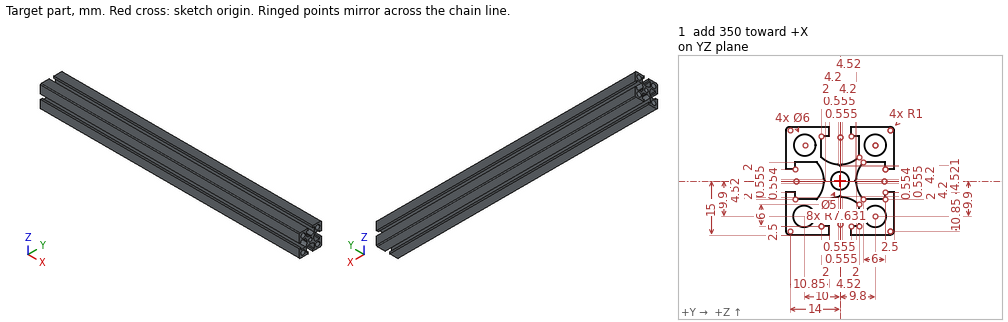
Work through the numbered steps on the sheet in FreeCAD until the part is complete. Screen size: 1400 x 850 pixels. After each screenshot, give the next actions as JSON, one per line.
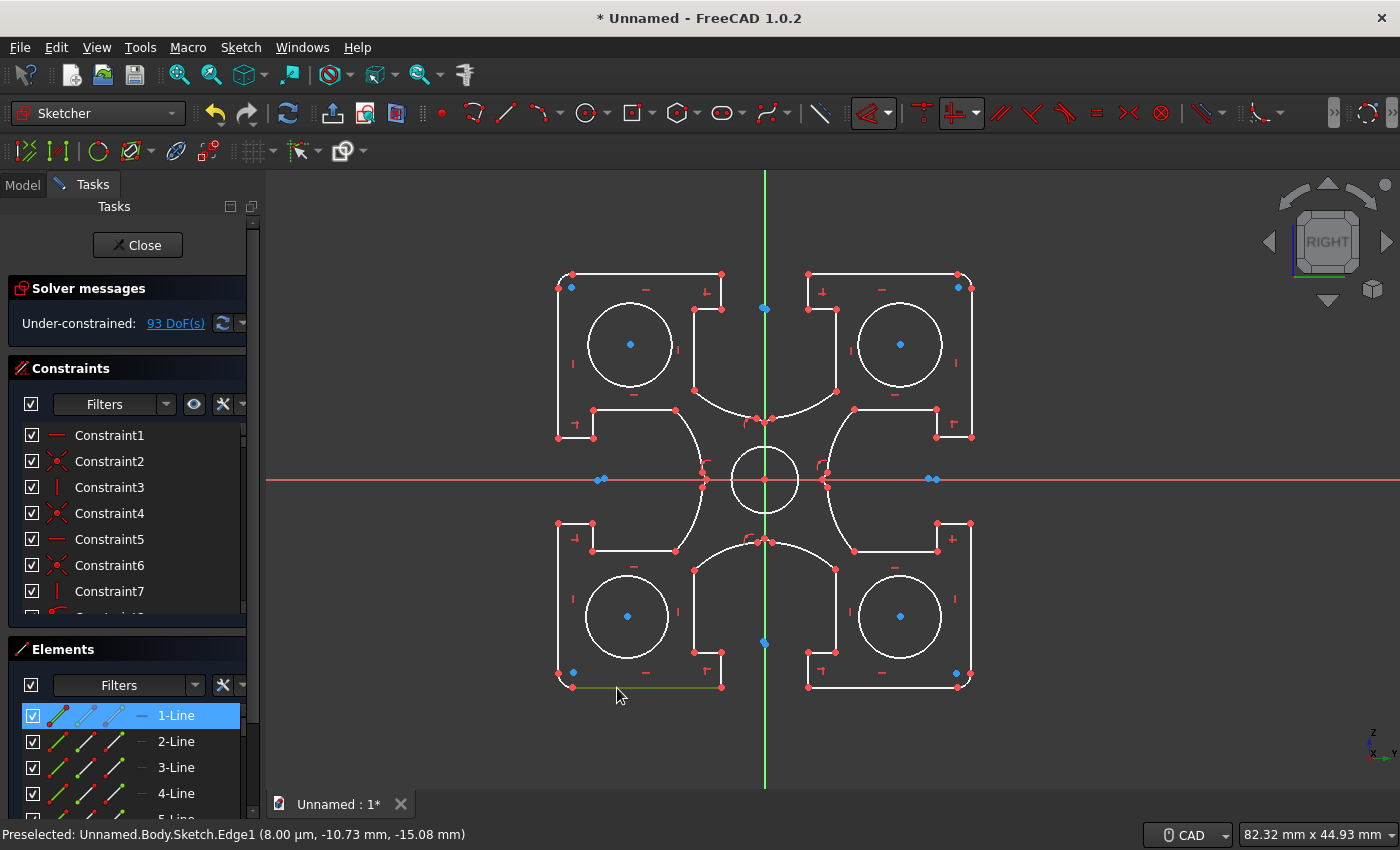
{"action": "scroll", "coordinate": [563, 683], "scroll_direction": "up", "scroll_amount": 2}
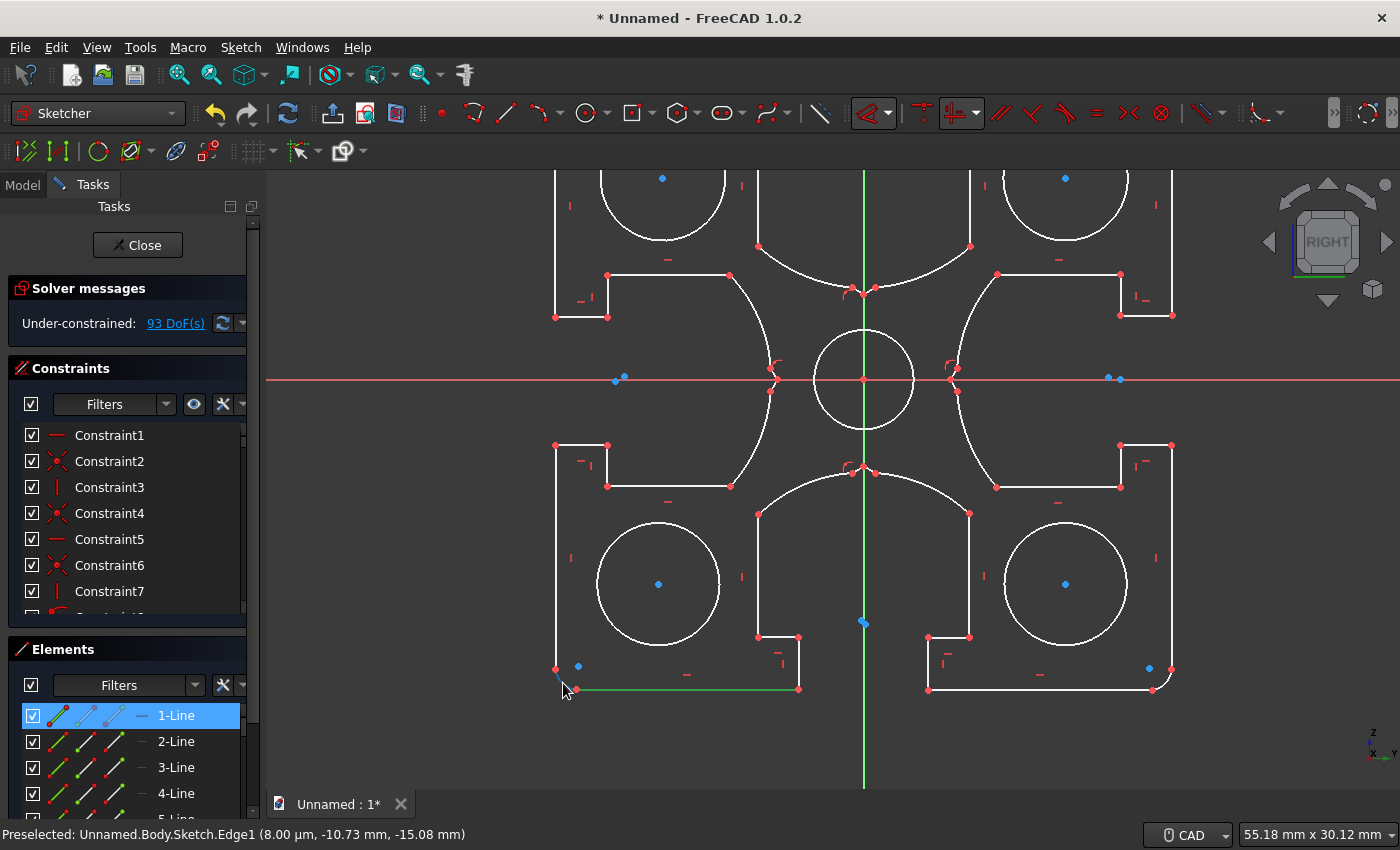
{"action": "left_click", "coordinate": [562, 683]}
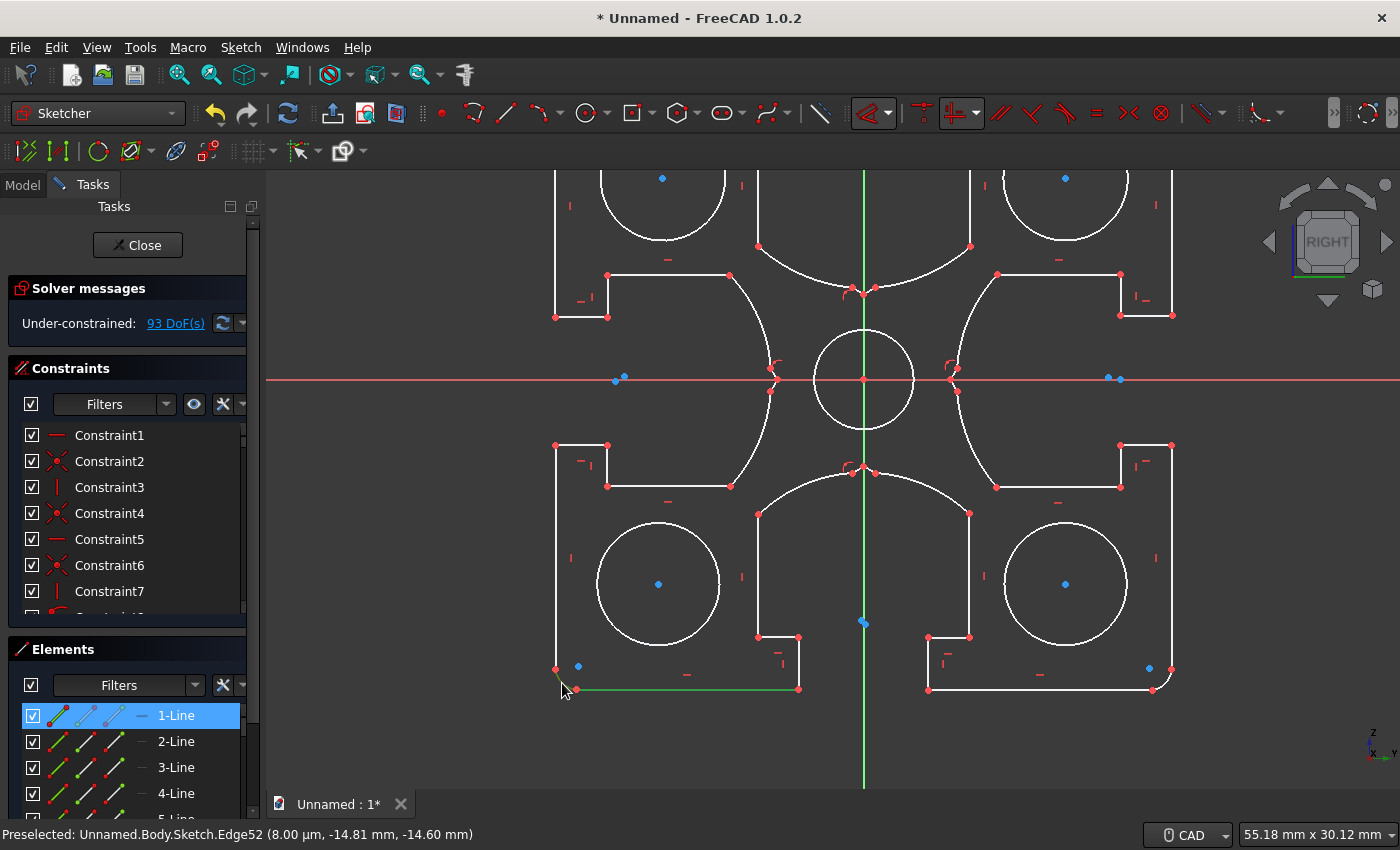
{"action": "left_click", "coordinate": [1066, 114]}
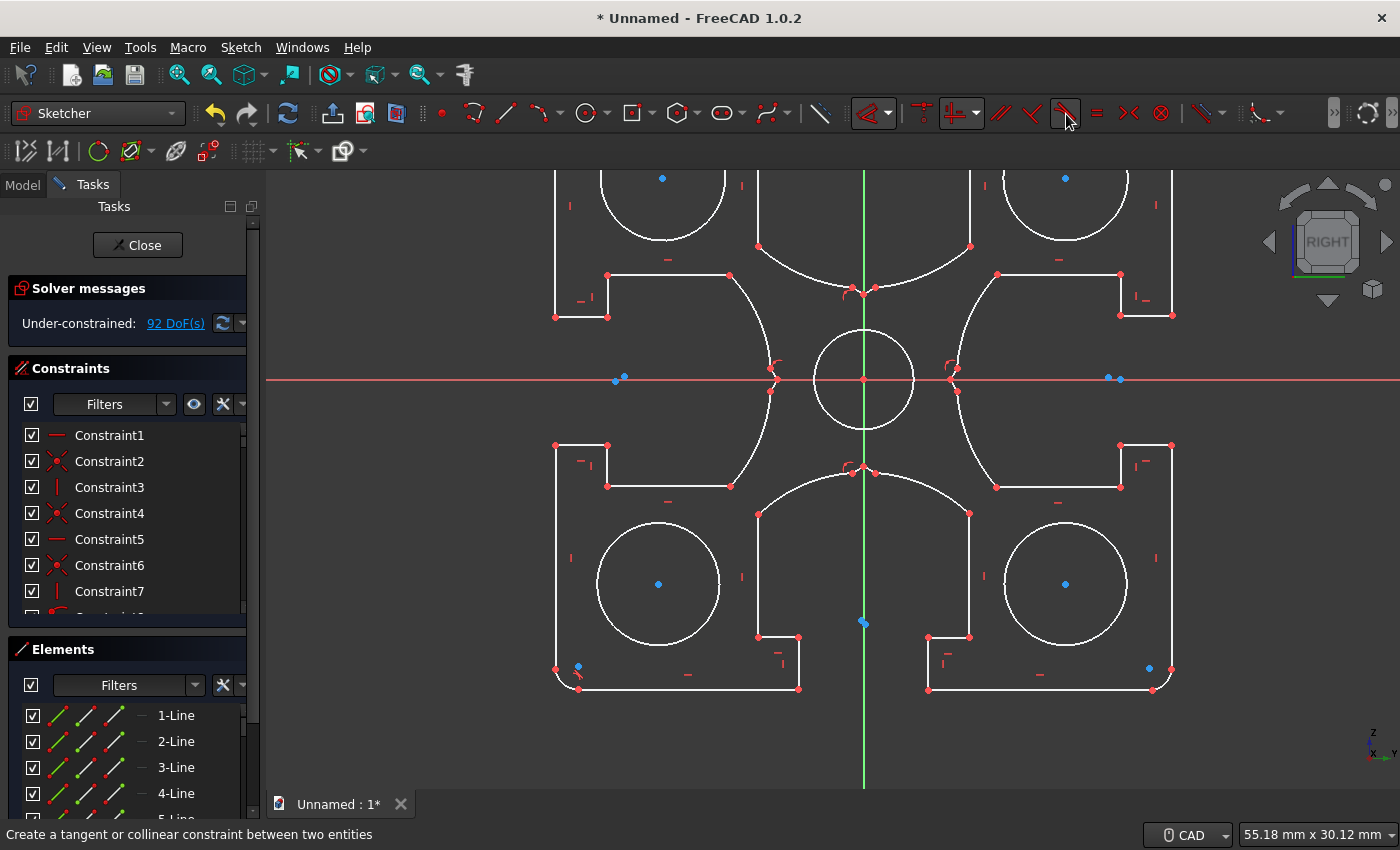
{"action": "left_click", "coordinate": [996, 690]}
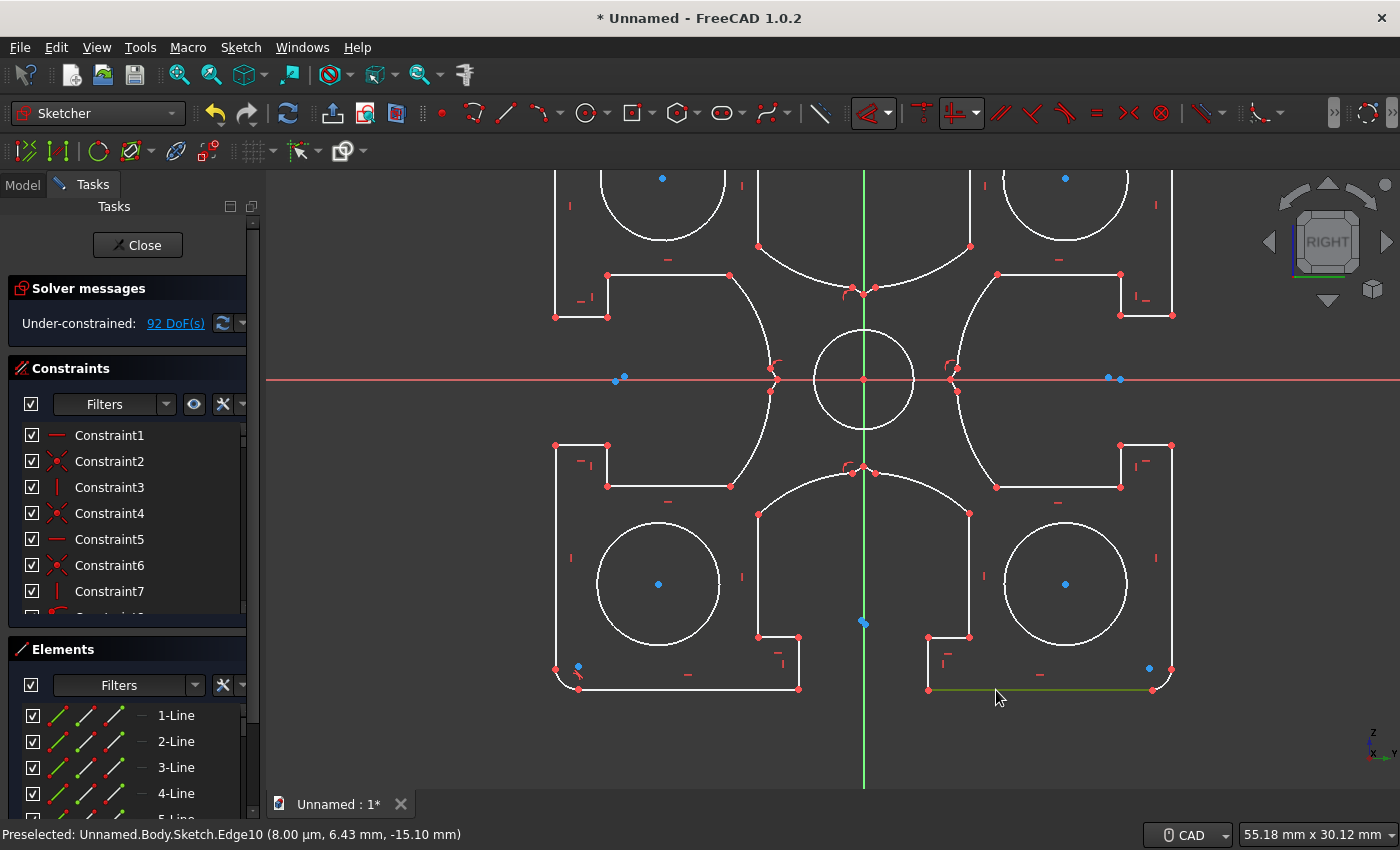
{"action": "scroll", "coordinate": [1161, 687], "scroll_direction": "up", "scroll_amount": 3}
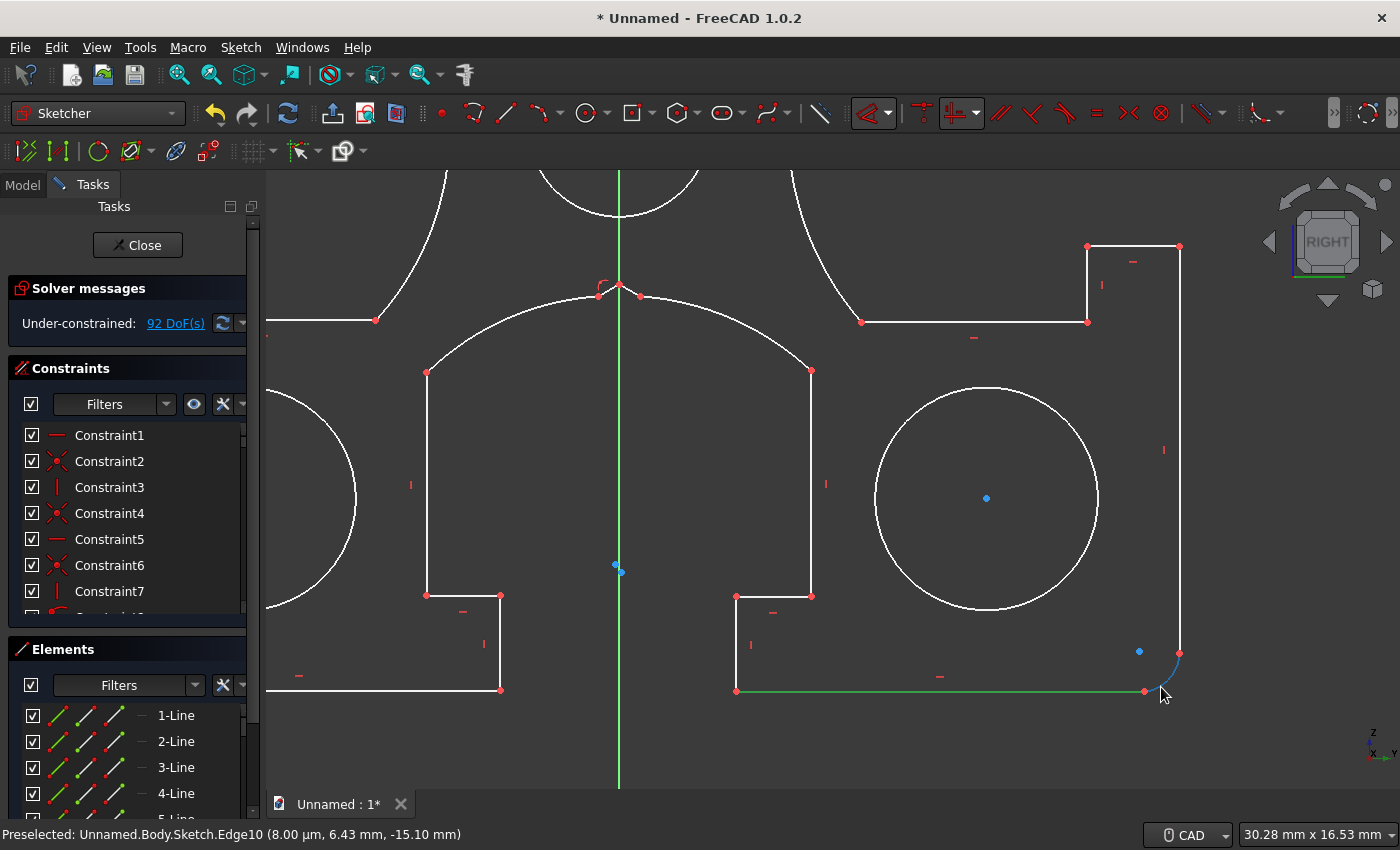
{"action": "left_click", "coordinate": [1160, 686]}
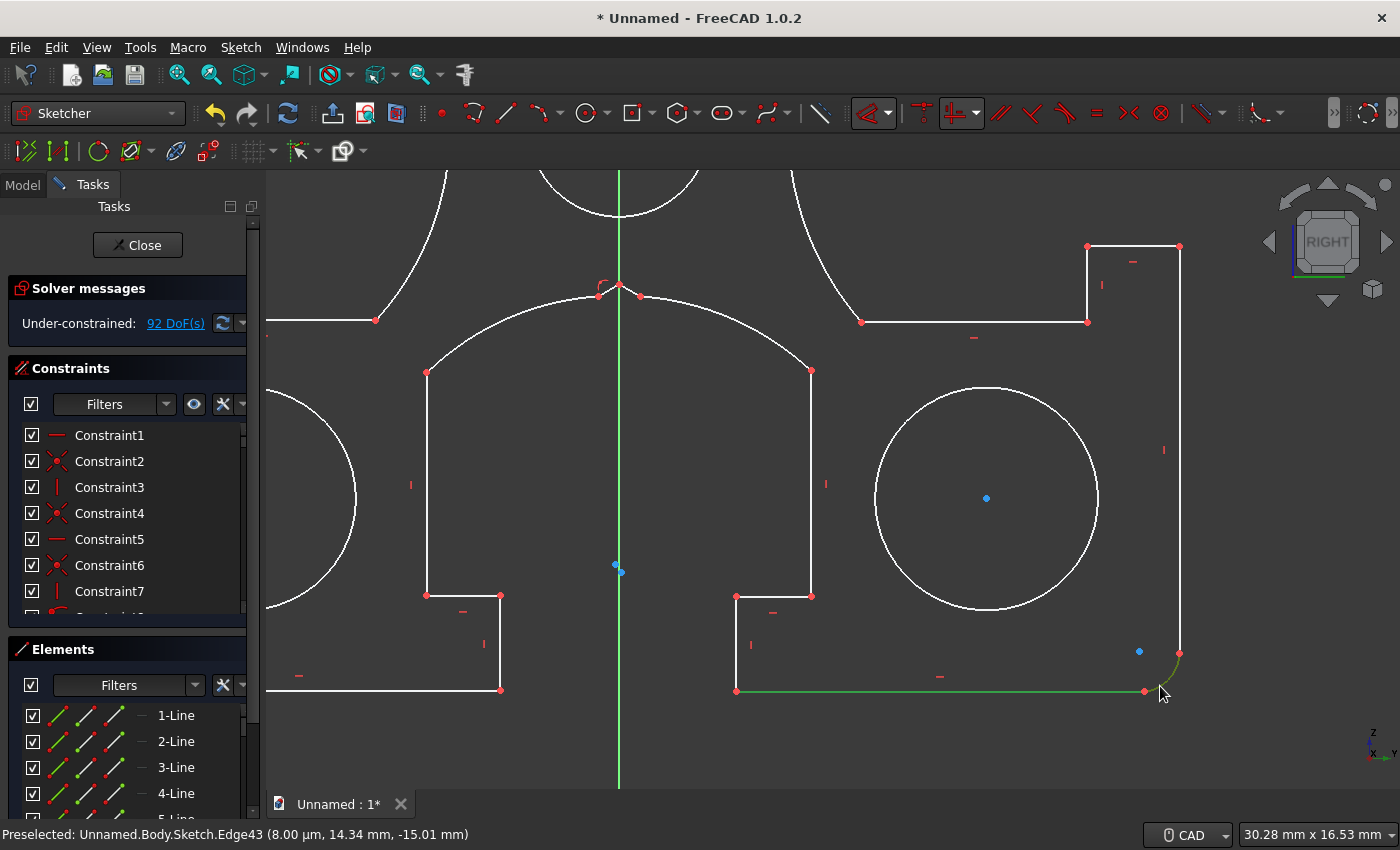
{"action": "left_click", "coordinate": [1066, 114]}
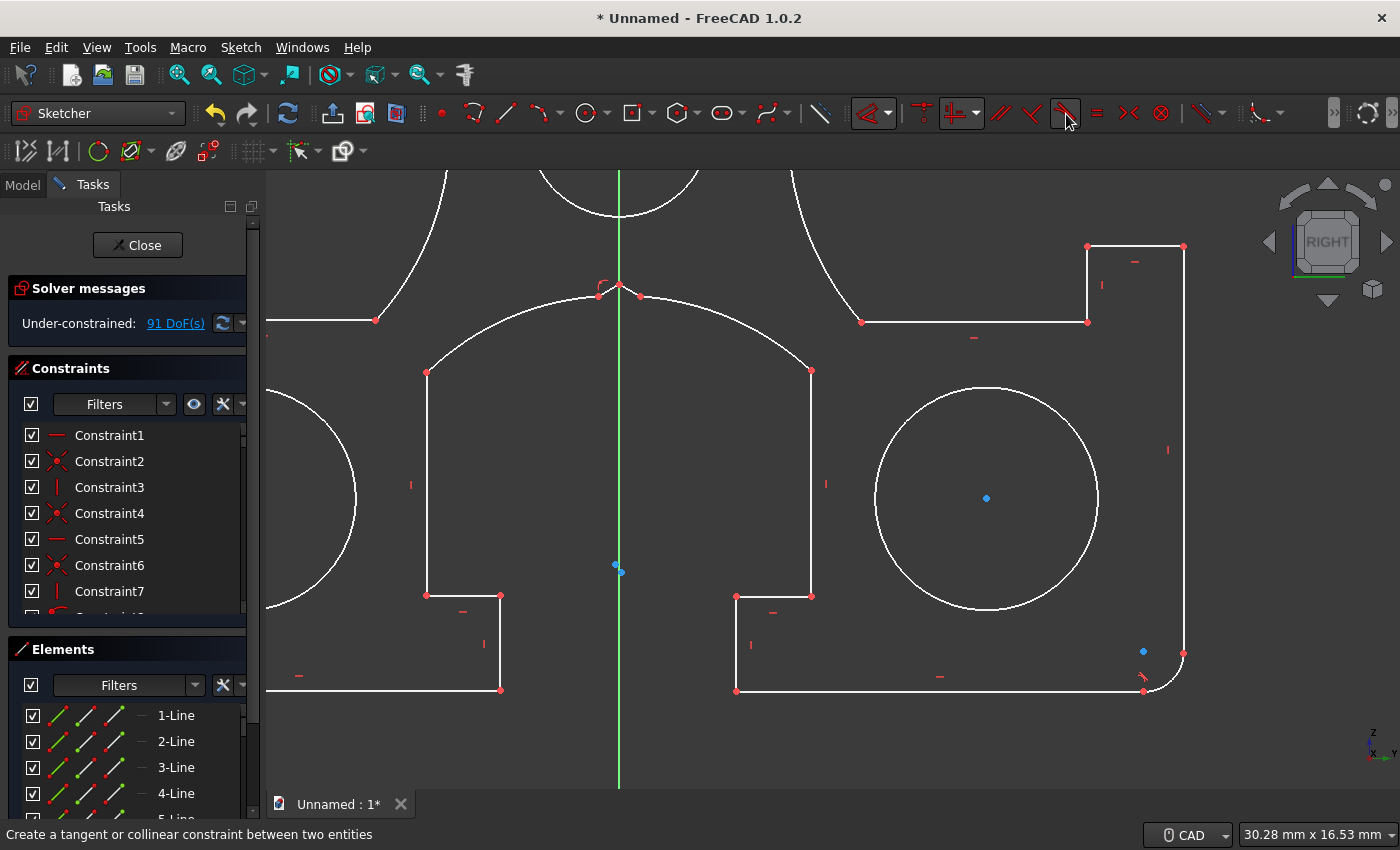
{"action": "left_click", "coordinate": [1184, 531]}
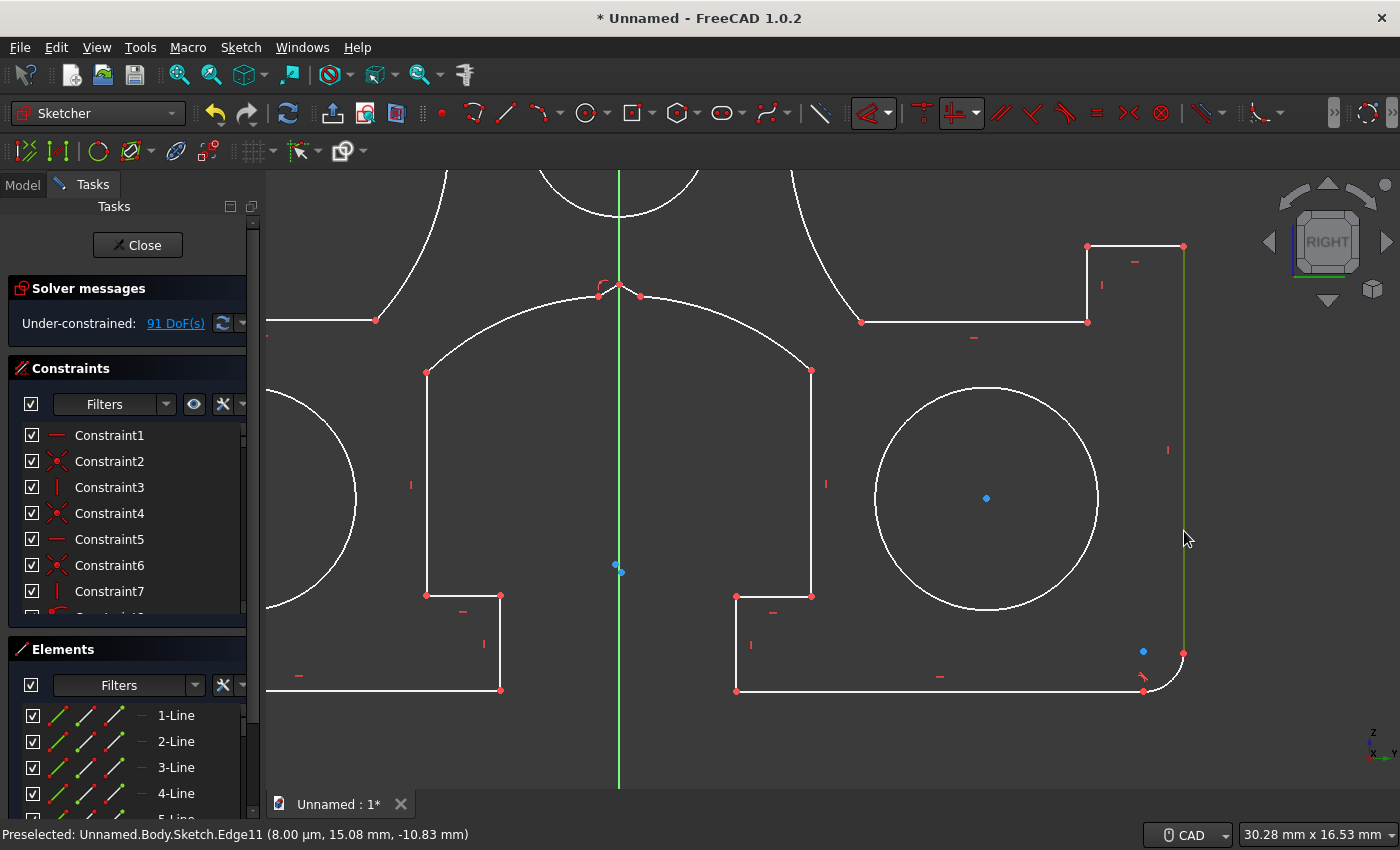
{"action": "left_click", "coordinate": [1161, 688]}